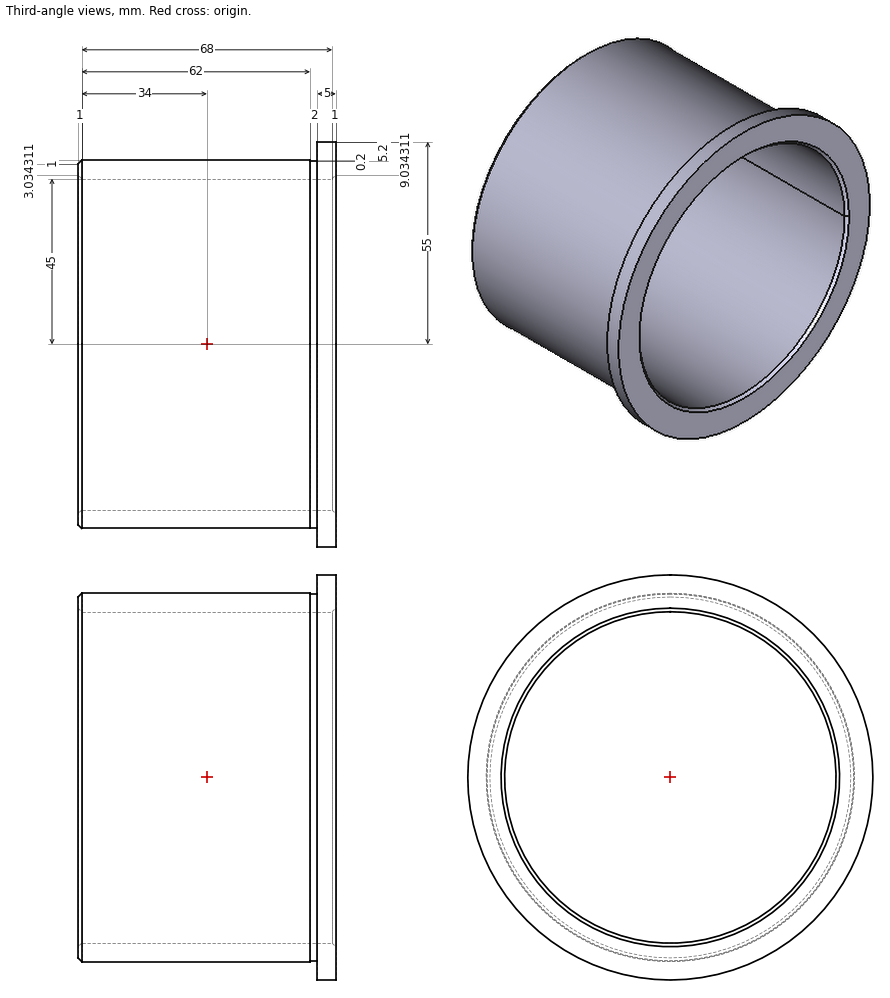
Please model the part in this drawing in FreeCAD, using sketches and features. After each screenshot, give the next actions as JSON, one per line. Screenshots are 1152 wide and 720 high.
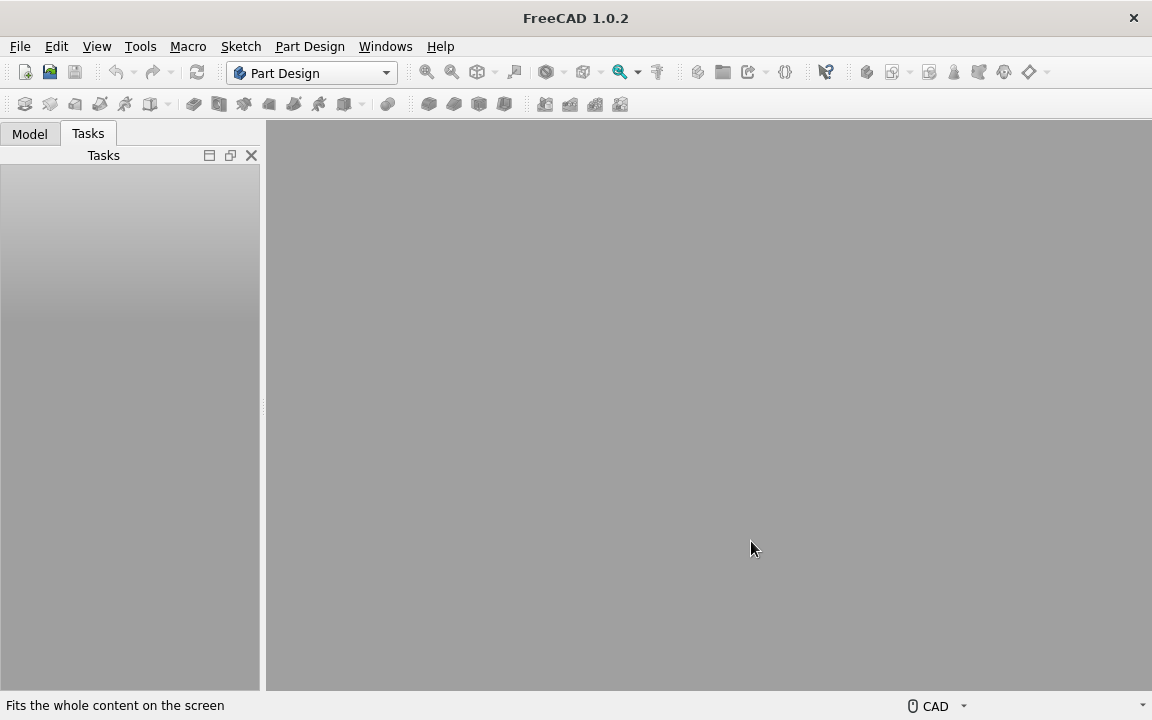
{"action": "left_click", "coordinate": [25, 72]}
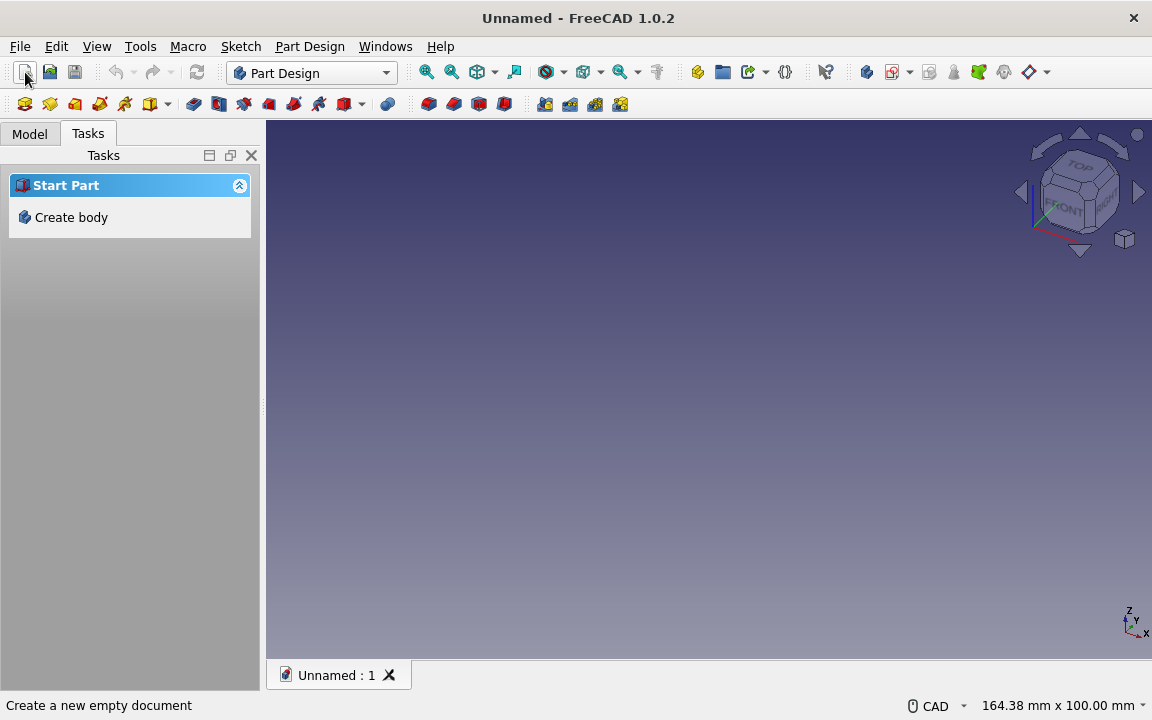
{"action": "left_click", "coordinate": [892, 72]}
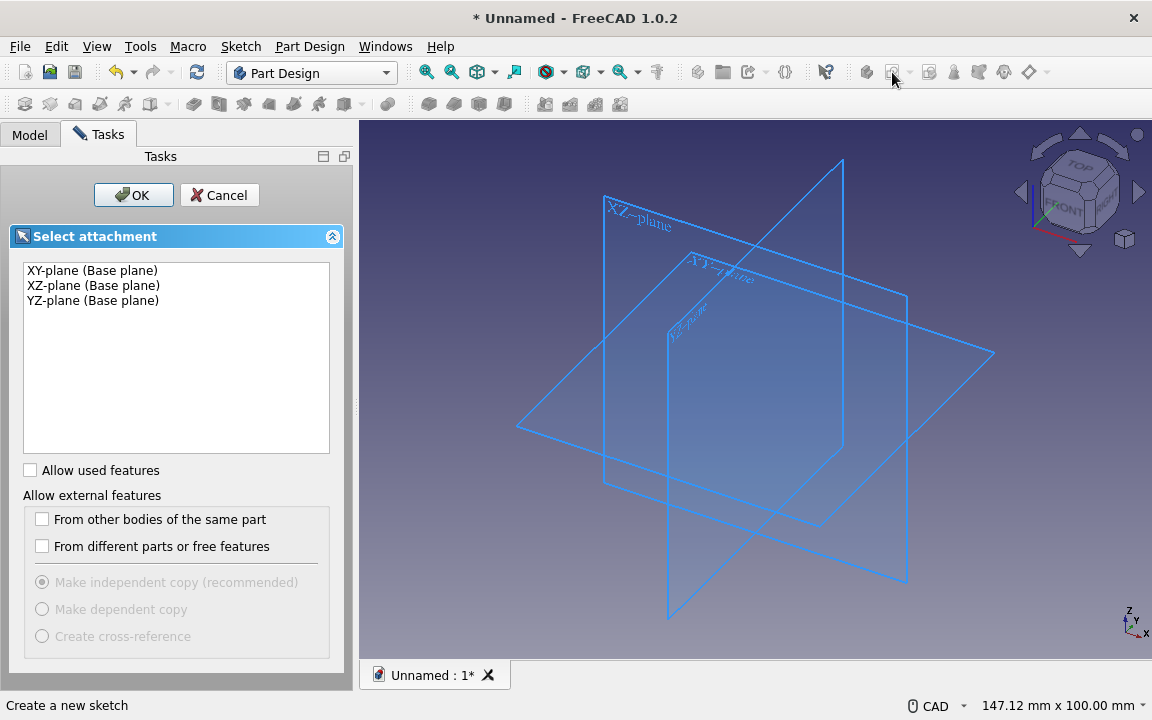
{"action": "left_click", "coordinate": [84, 270]}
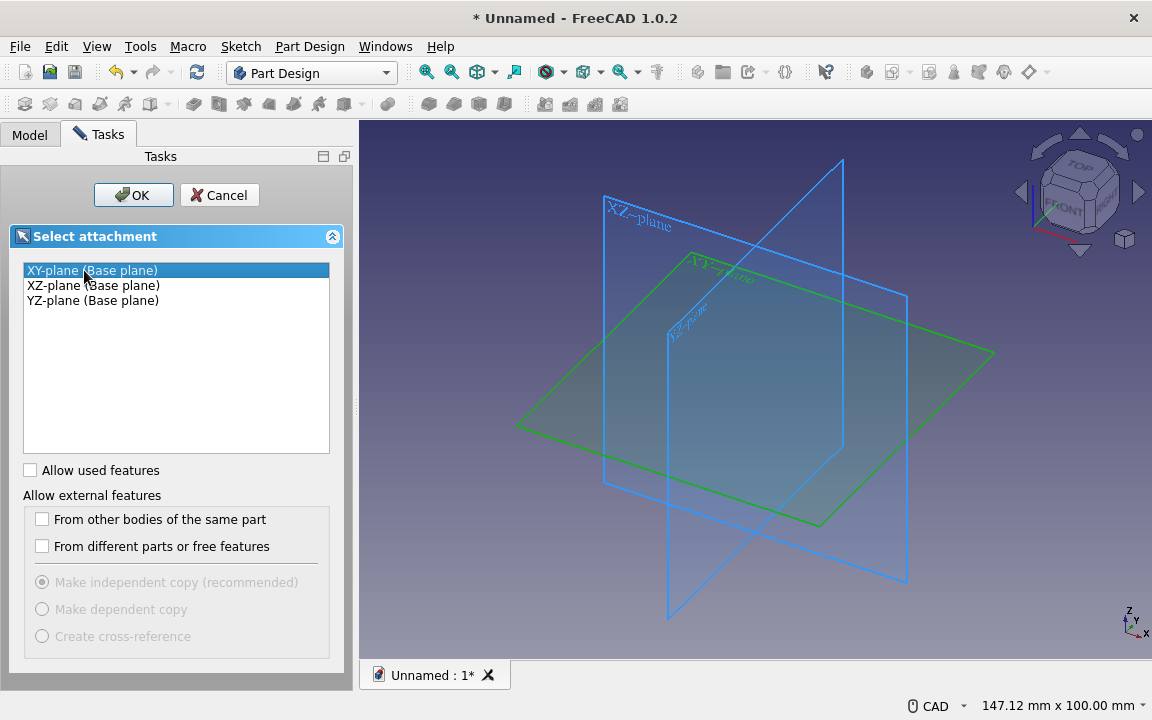
{"action": "left_click", "coordinate": [134, 195]}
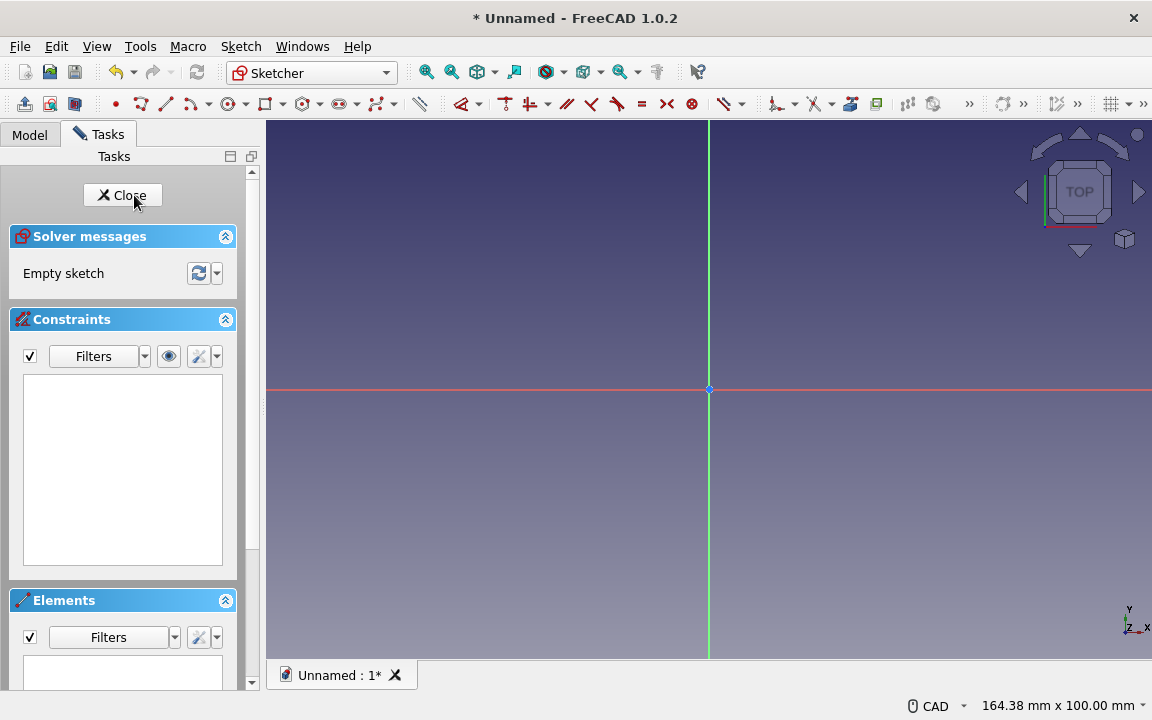
{"action": "scroll", "coordinate": [331, 631], "scroll_direction": "down", "scroll_amount": 1}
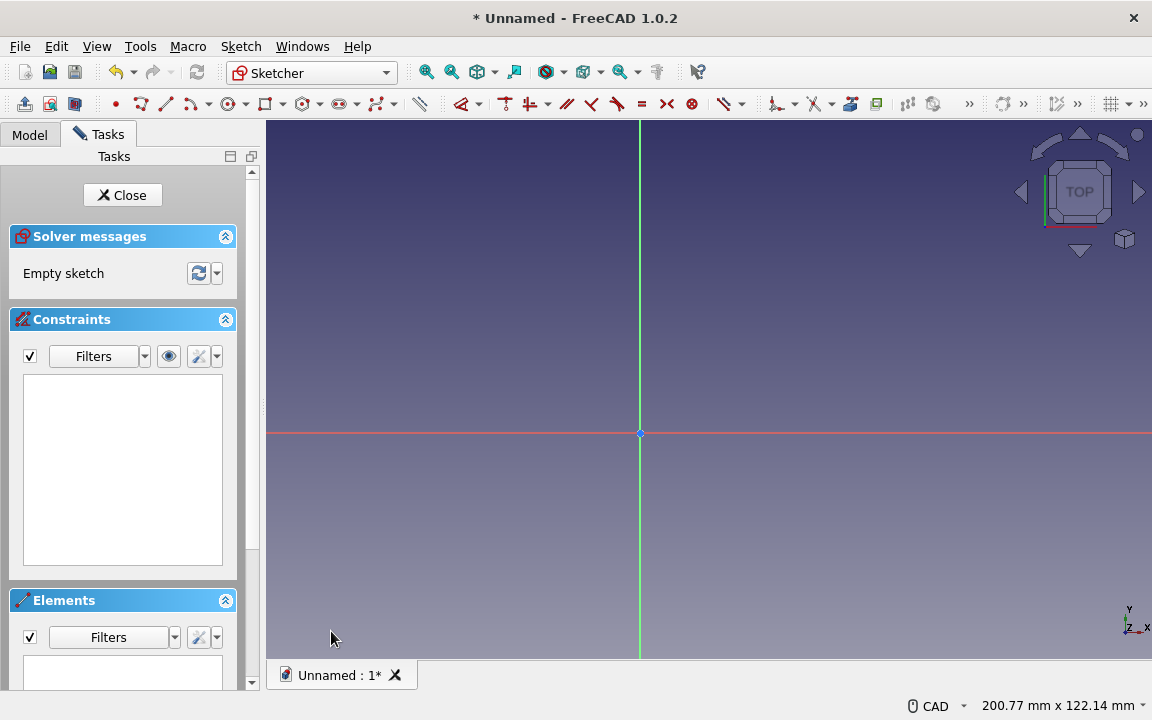
{"action": "scroll", "coordinate": [640, 155], "scroll_direction": "up", "scroll_amount": 2}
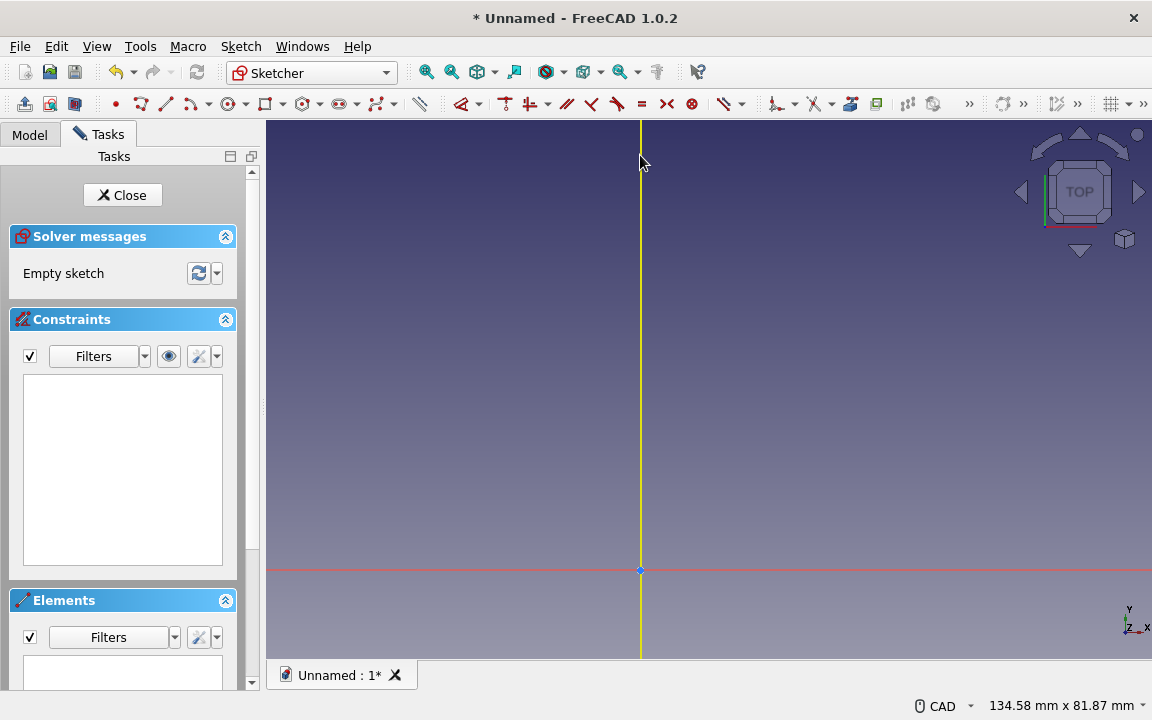
{"action": "key", "text": "g m"}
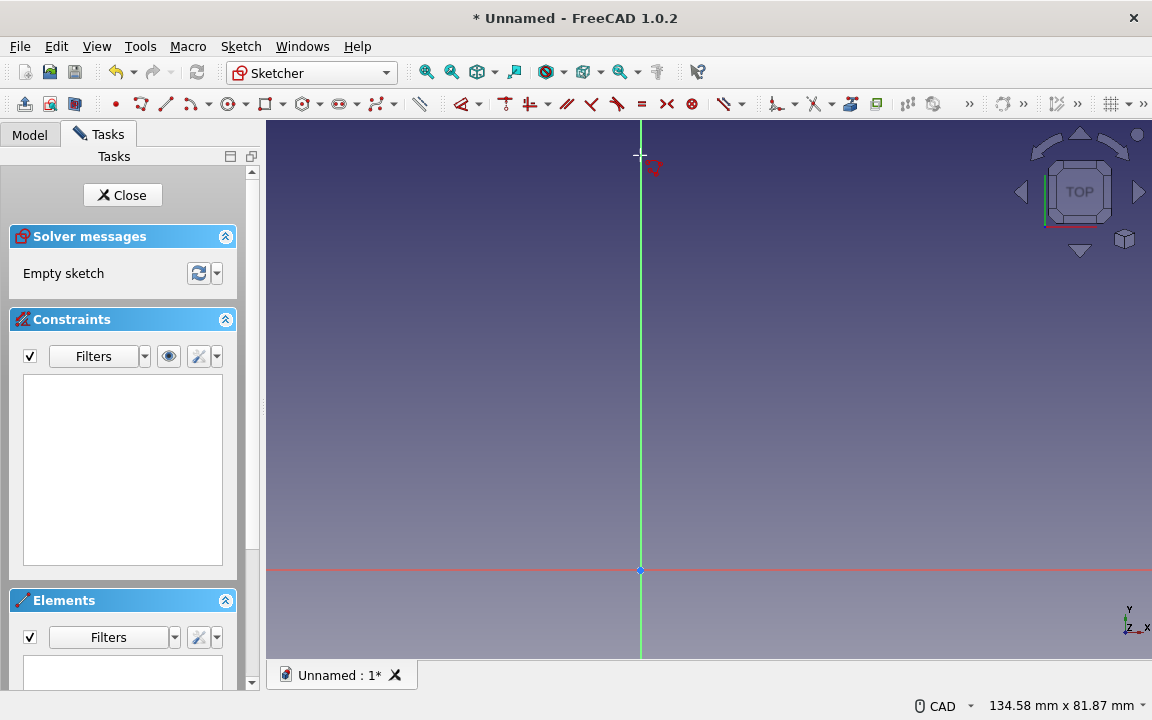
{"action": "left_click", "coordinate": [417, 274]}
{"action": "left_click", "coordinate": [864, 274]}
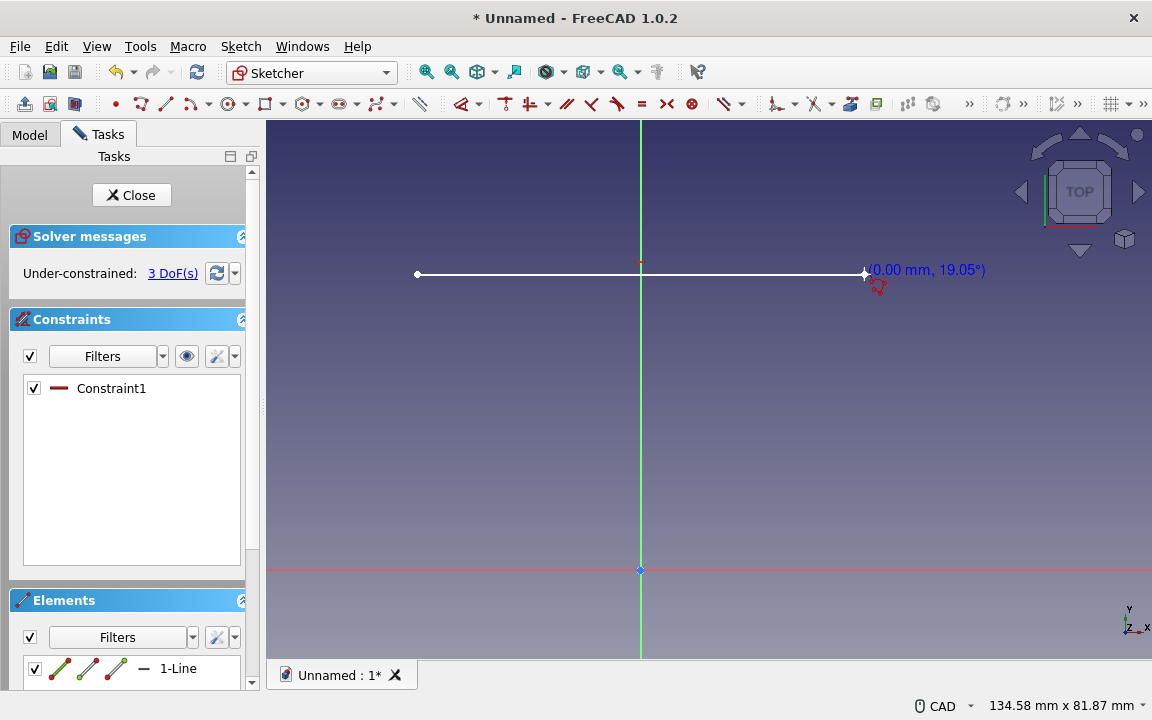
{"action": "scroll", "coordinate": [871, 268], "scroll_direction": "up", "scroll_amount": 3}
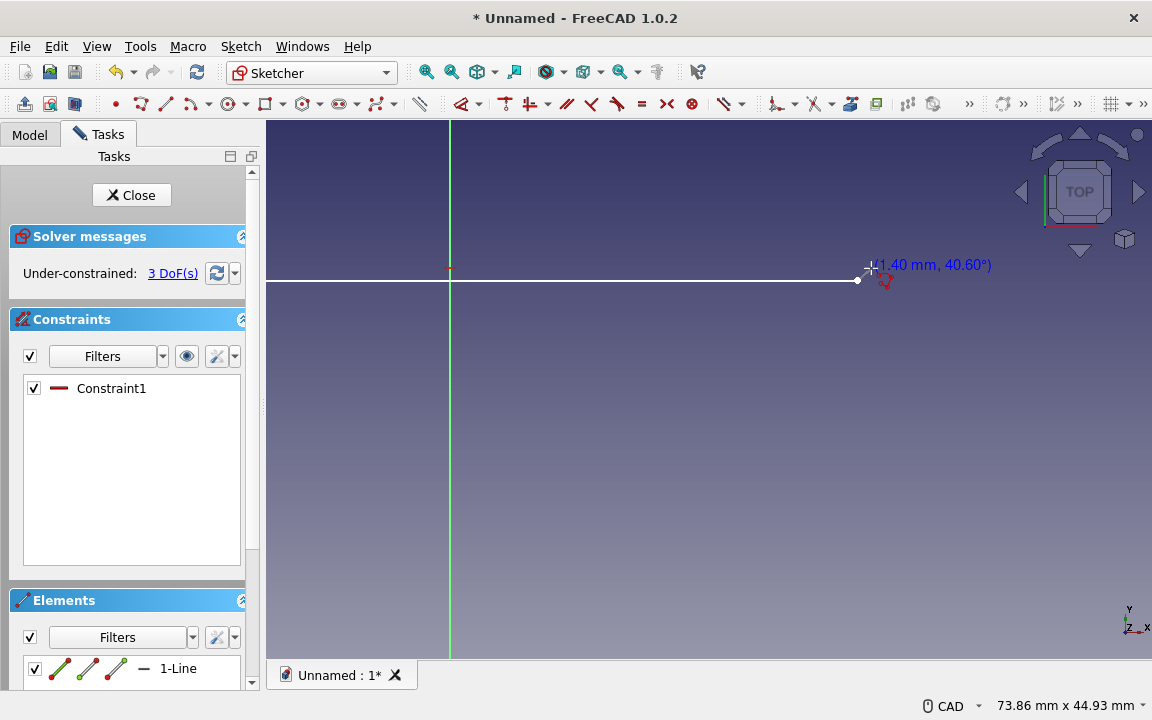
{"action": "left_click", "coordinate": [870, 267]}
{"action": "left_click", "coordinate": [870, 159]}
{"action": "left_click", "coordinate": [810, 159]}
{"action": "left_click", "coordinate": [810, 221]}
{"action": "left_click", "coordinate": [786, 221]}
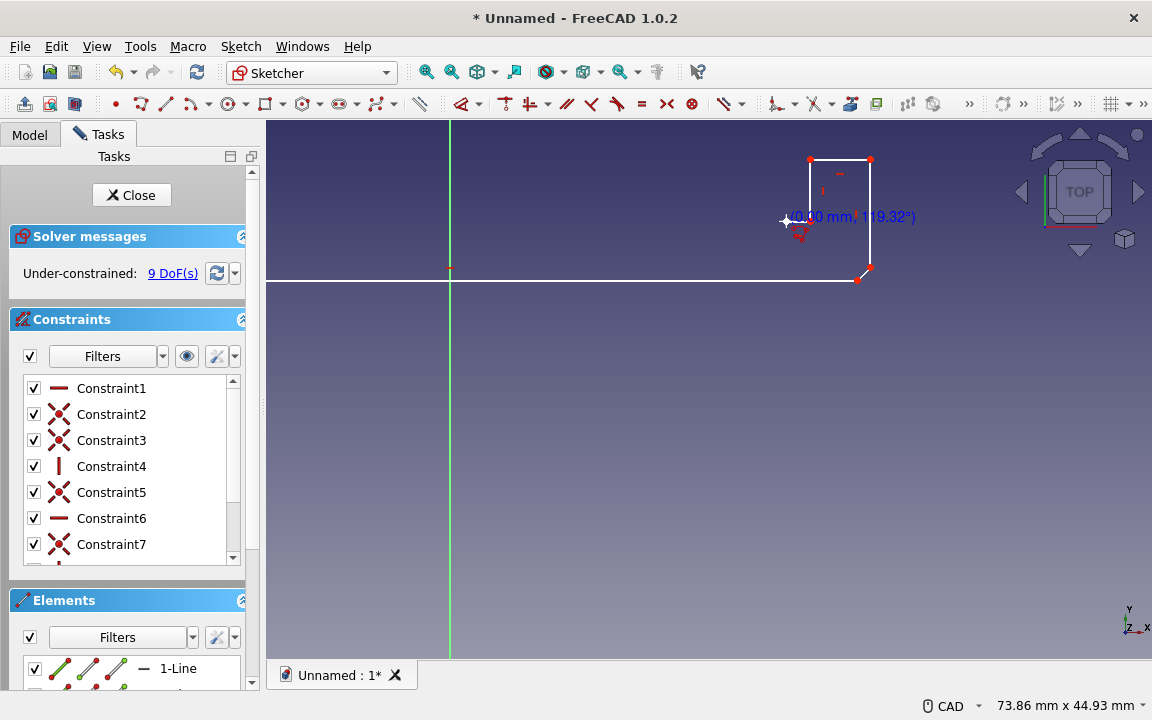
{"action": "scroll", "coordinate": [786, 219], "scroll_direction": "up", "scroll_amount": 10}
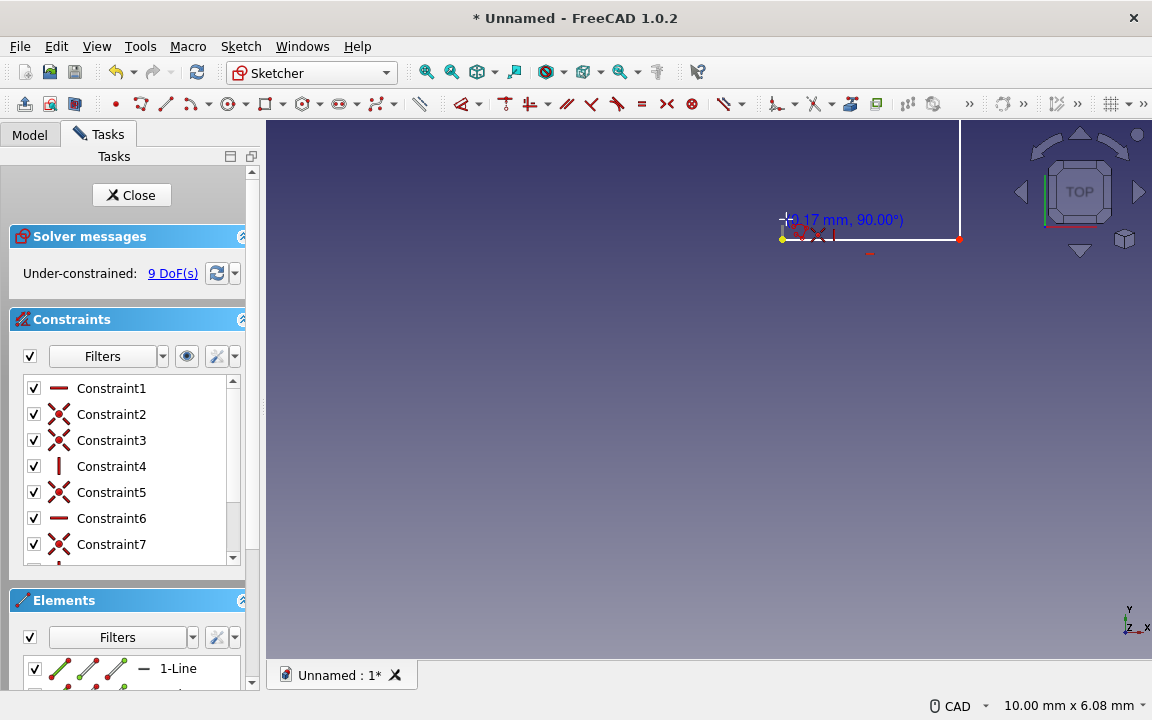
{"action": "left_click", "coordinate": [782, 217]}